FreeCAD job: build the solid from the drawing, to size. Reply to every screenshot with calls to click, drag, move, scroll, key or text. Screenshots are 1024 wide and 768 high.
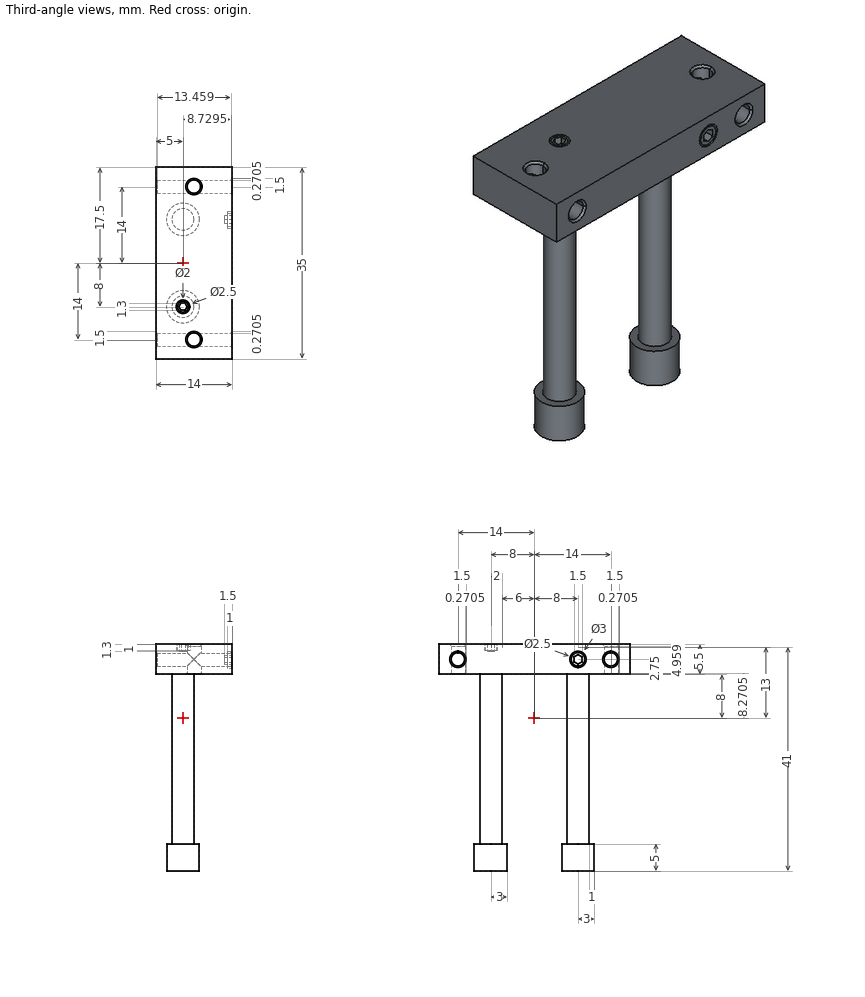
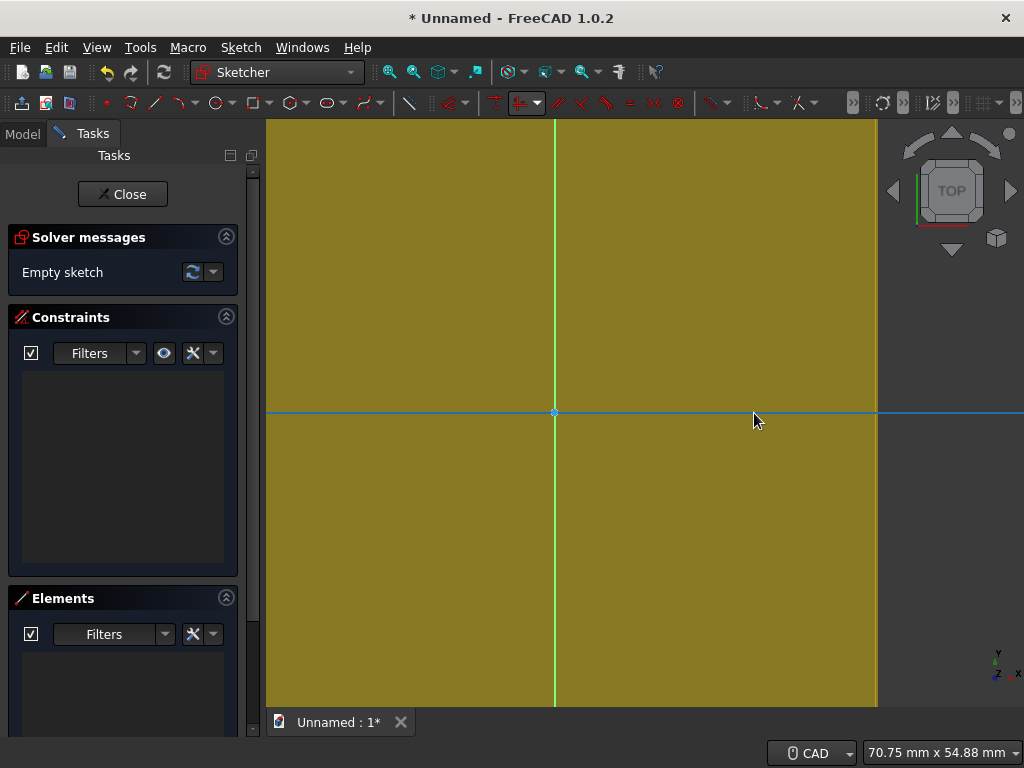
click(254, 104)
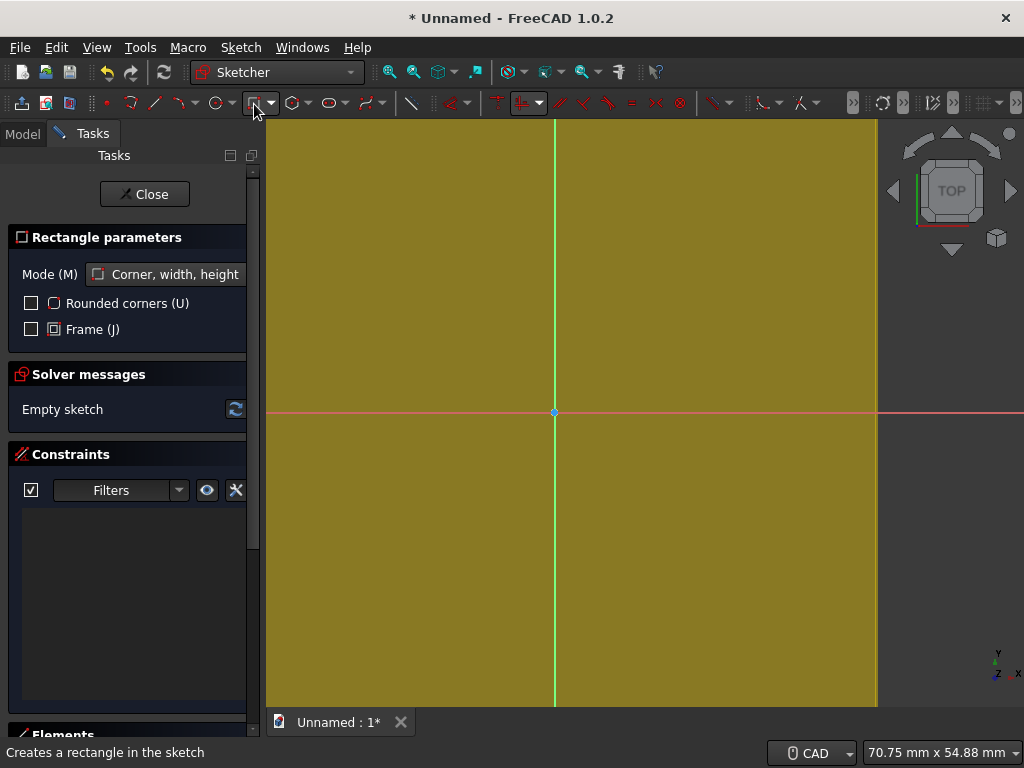
click(501, 225)
move(651, 600)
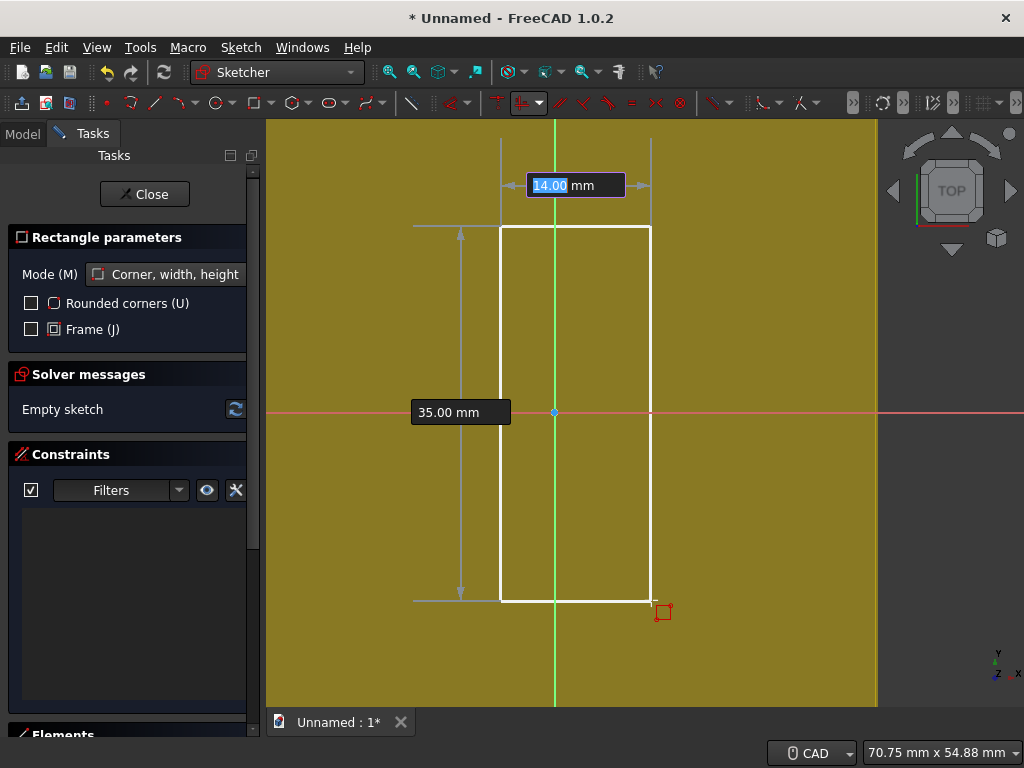
text(14)
key(Tab)
text(35)
key(Return)
key(Escape)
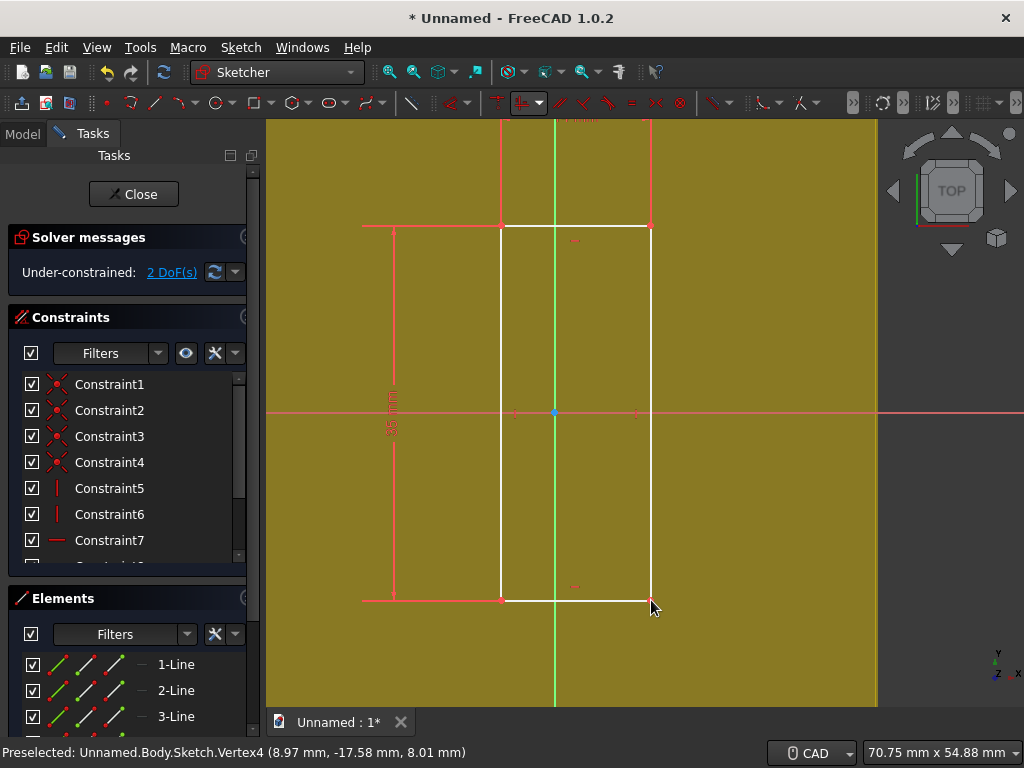
click(450, 104)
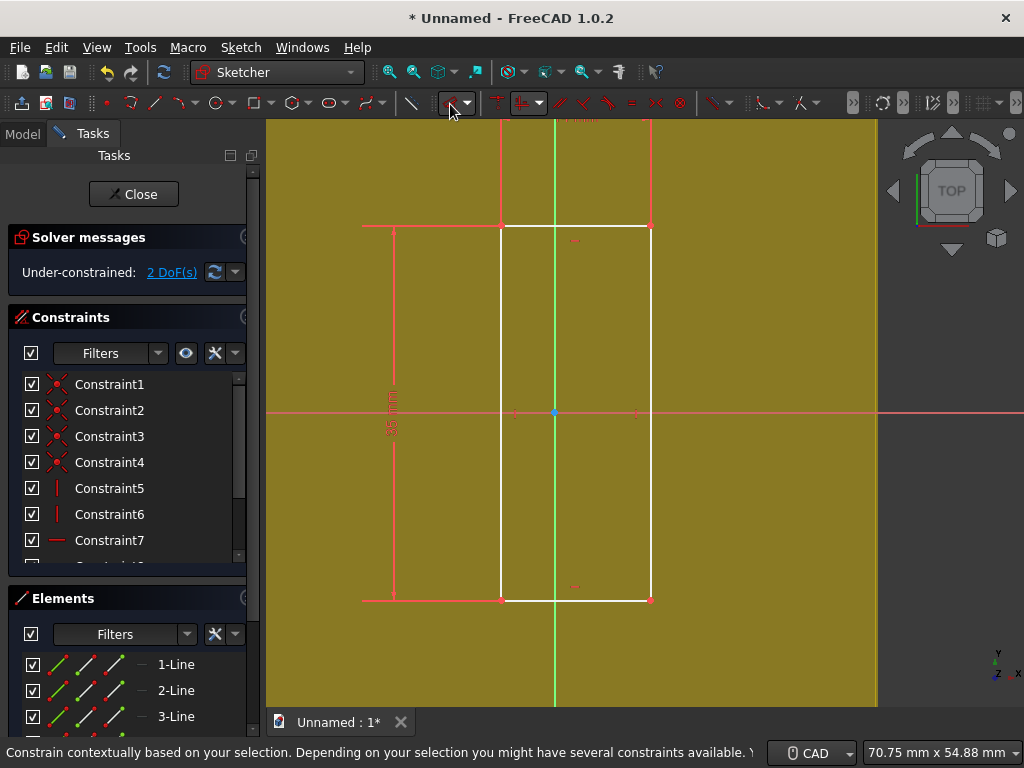
click(501, 226)
click(528, 192)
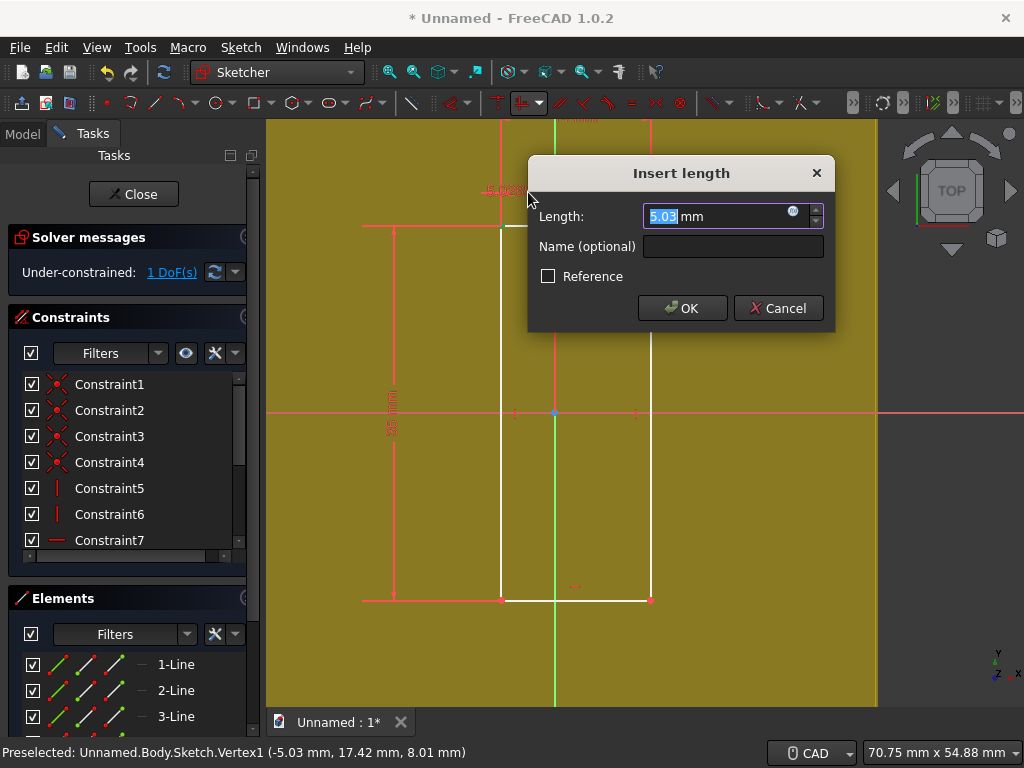
text(5)
key(Return)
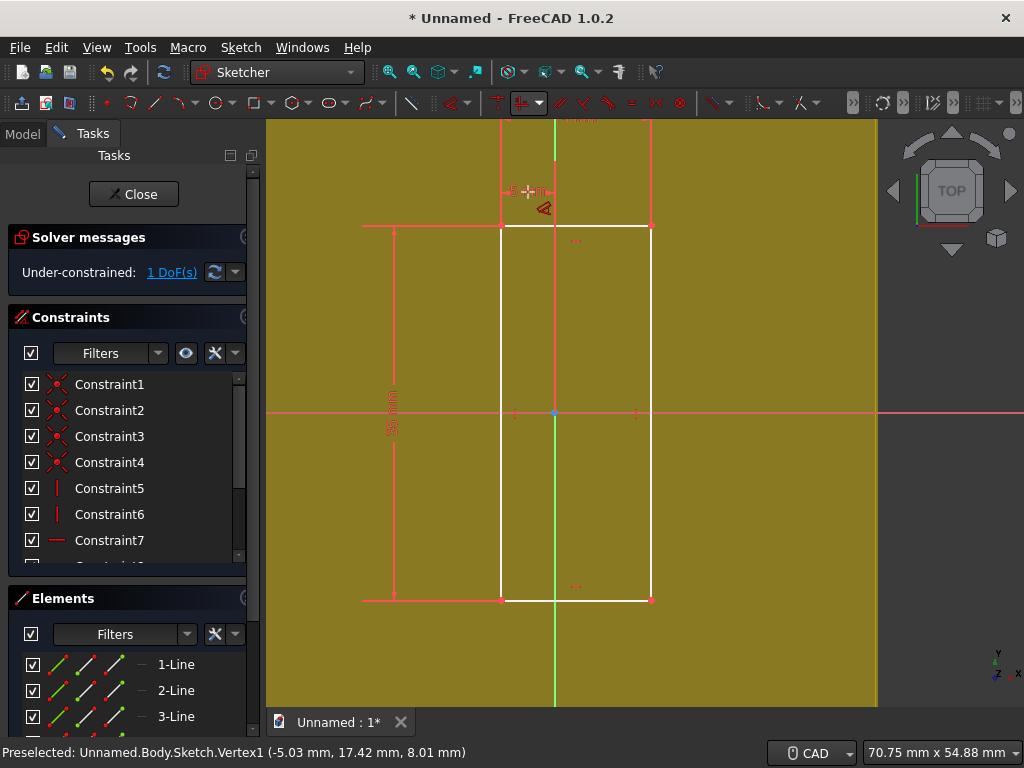
click(501, 226)
click(467, 319)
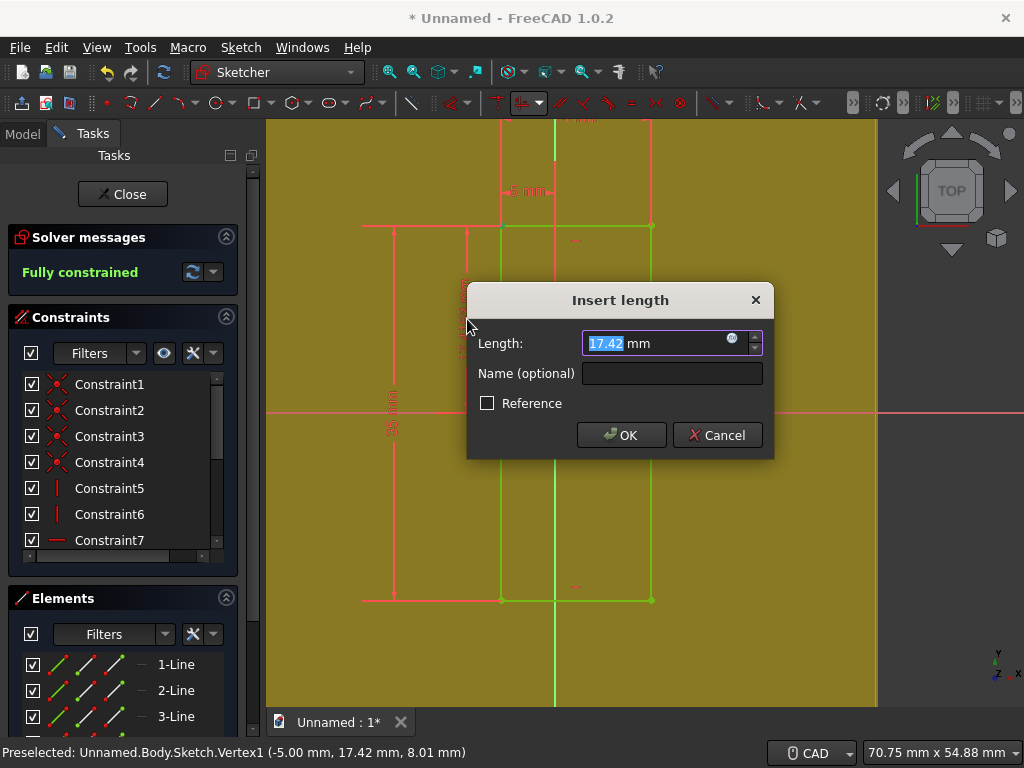
text(17.5)
key(Return)
key(Escape)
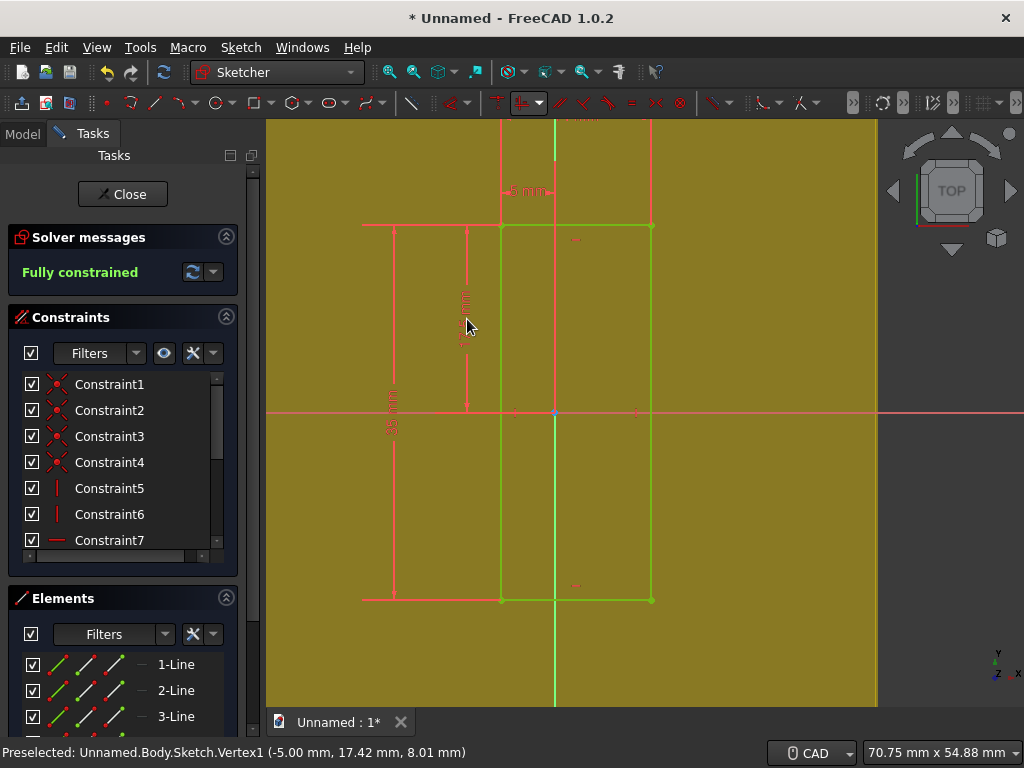
click(123, 194)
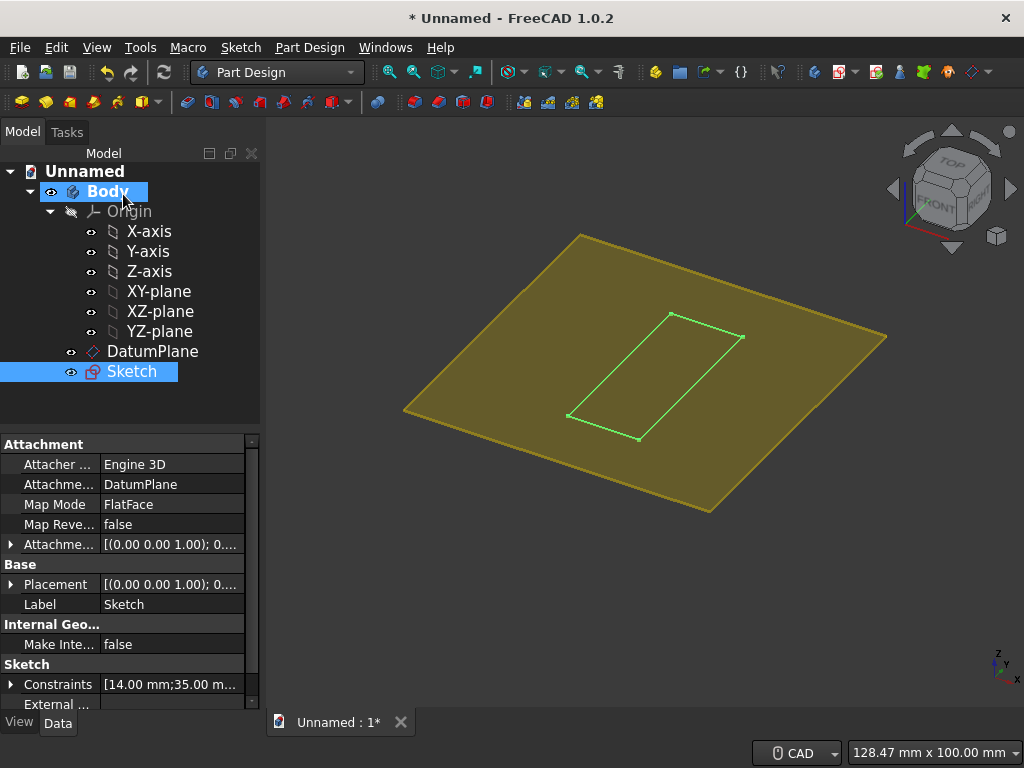
click(22, 102)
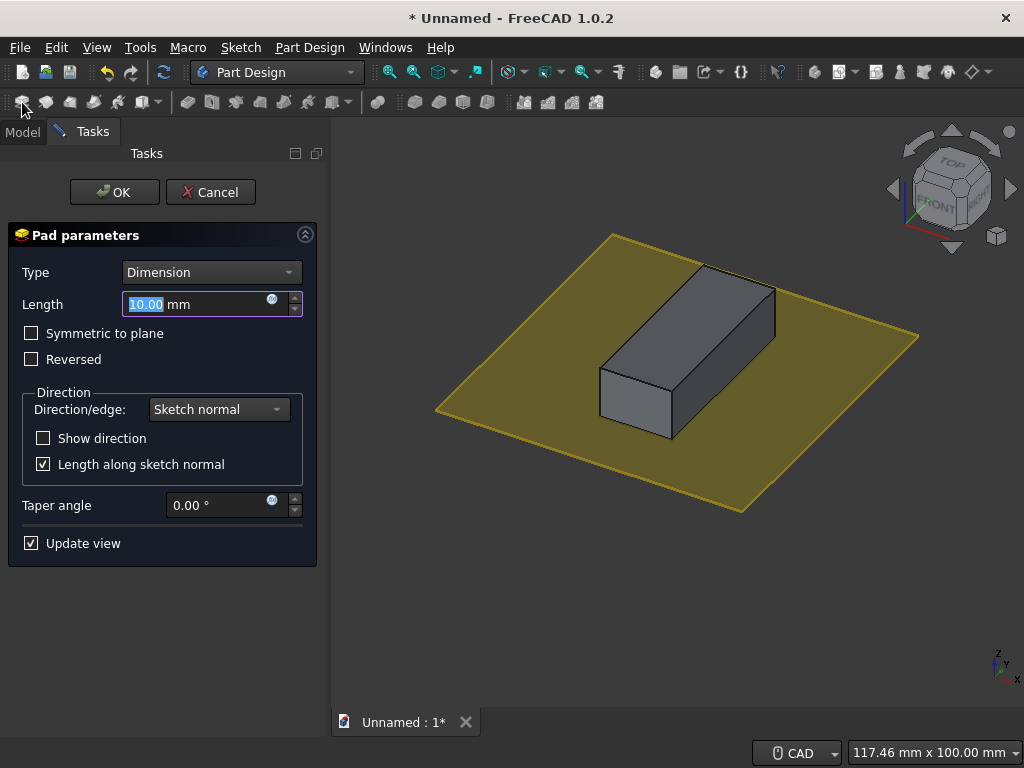
text(5.5)
key(Tab)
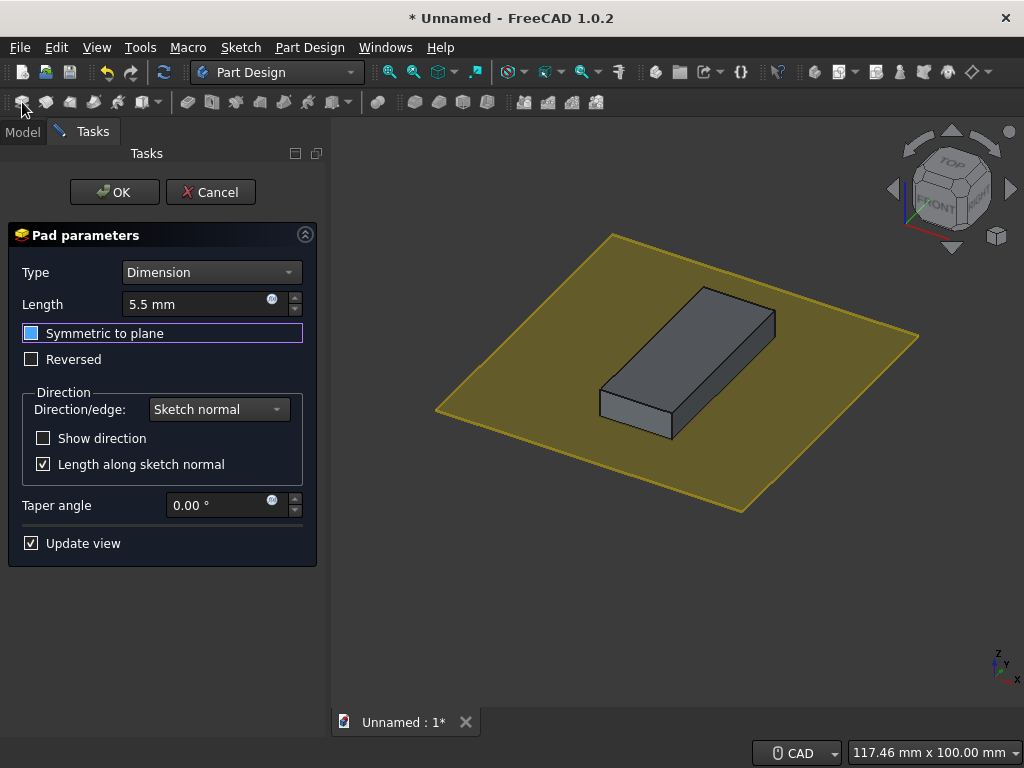
click(115, 192)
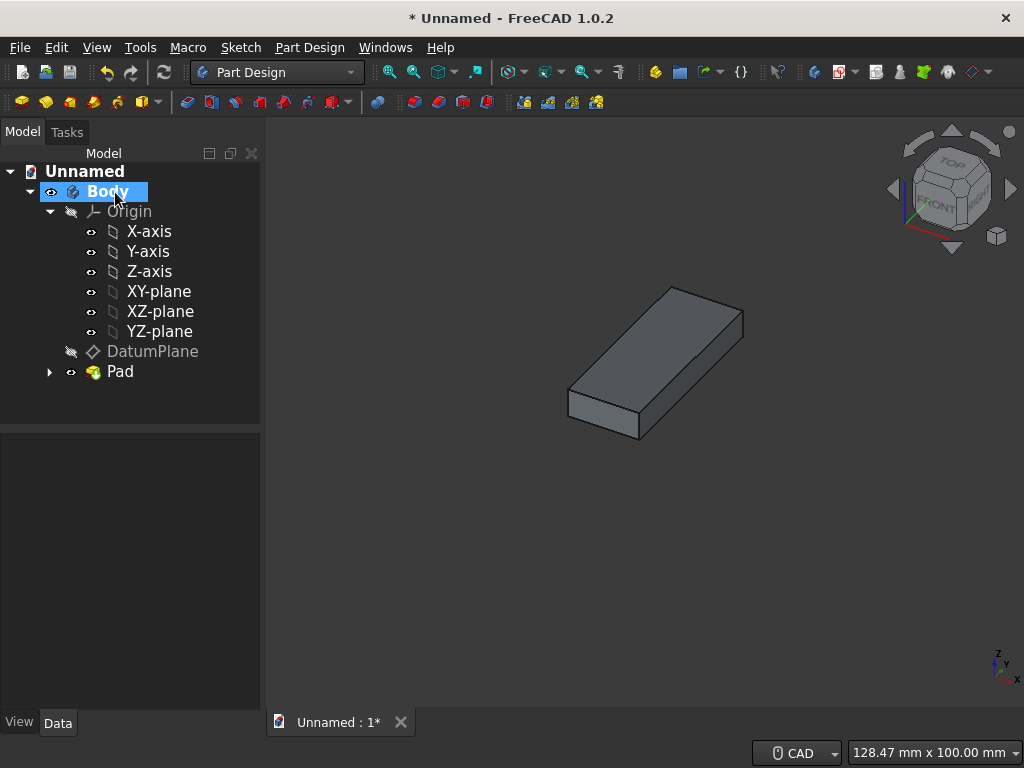
click(390, 72)